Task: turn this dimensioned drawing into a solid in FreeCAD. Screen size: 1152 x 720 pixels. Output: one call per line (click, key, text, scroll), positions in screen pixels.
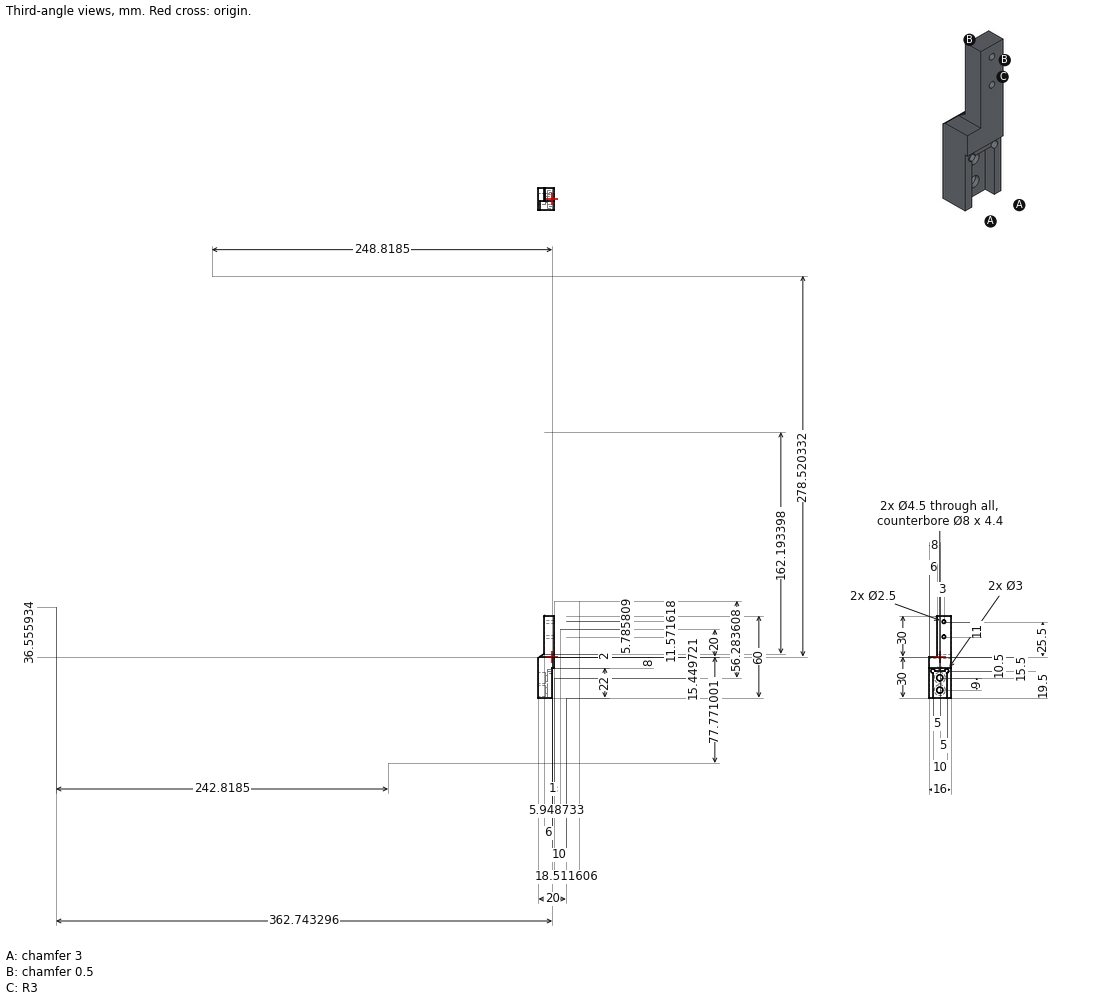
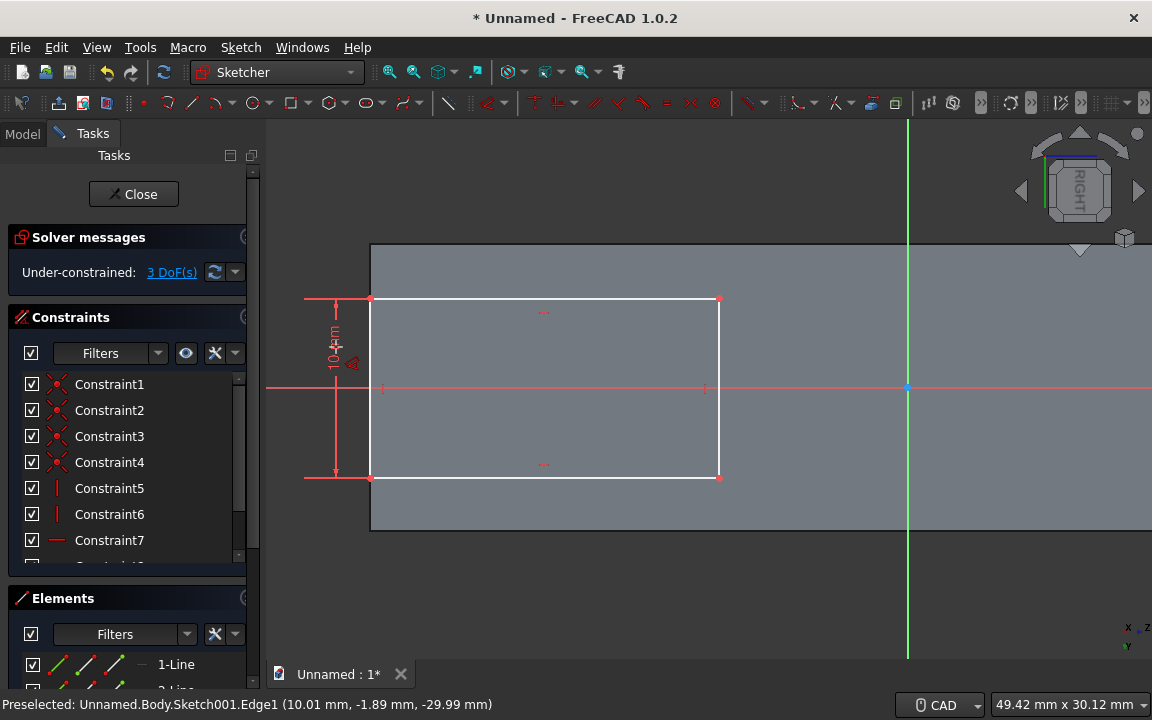
click(370, 299)
click(942, 343)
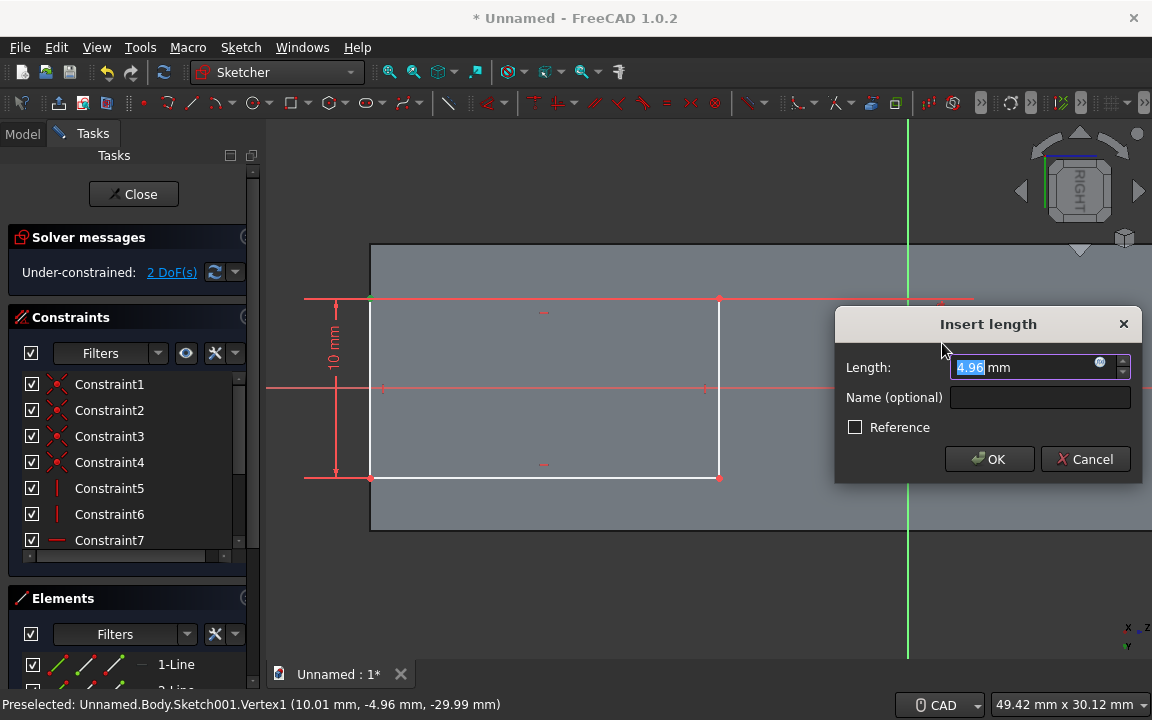
text(5)
key(Return)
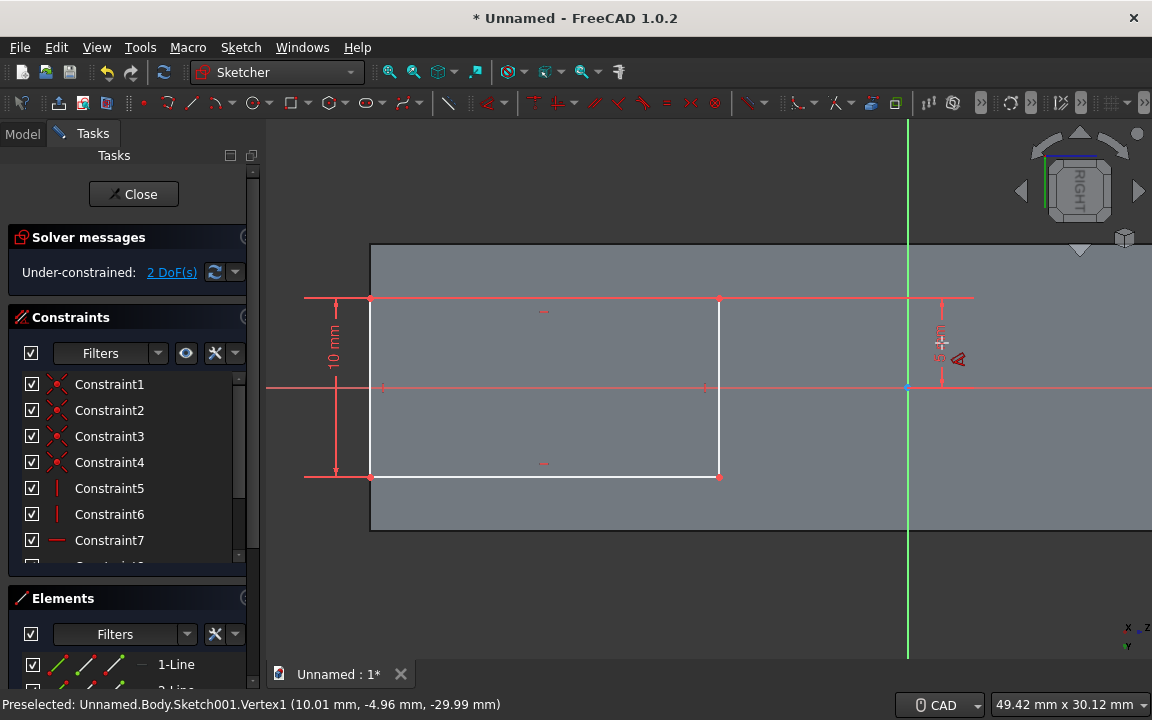
click(370, 298)
click(639, 264)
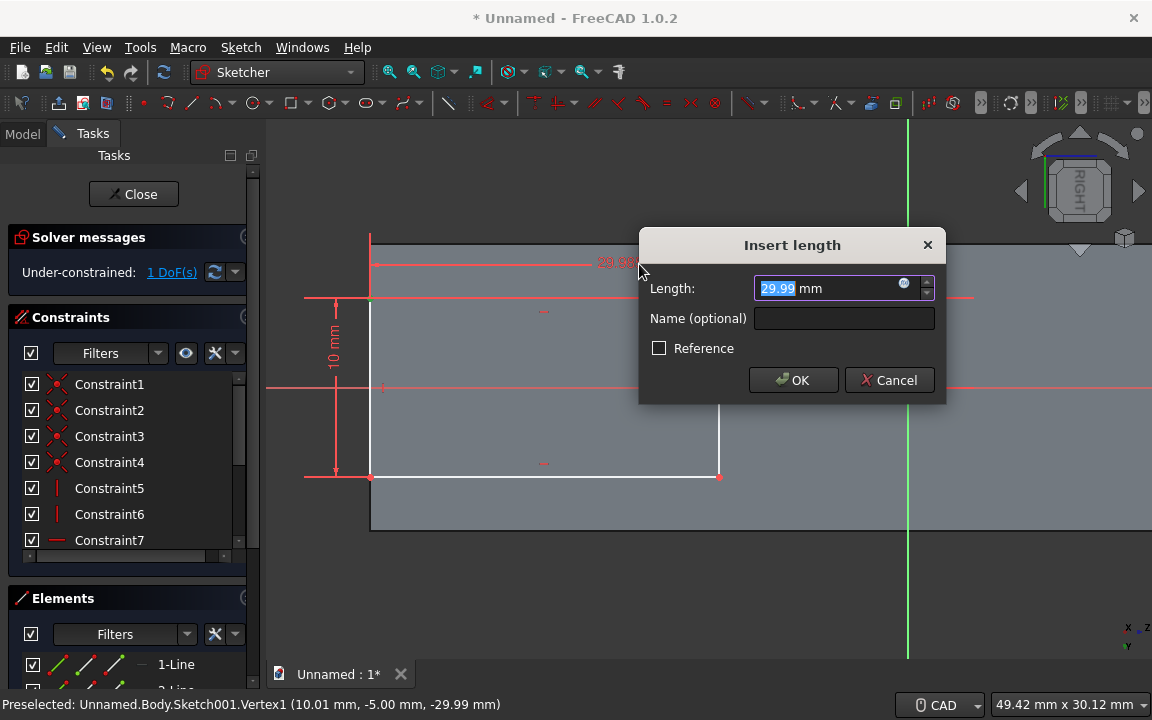
text(30)
key(Return)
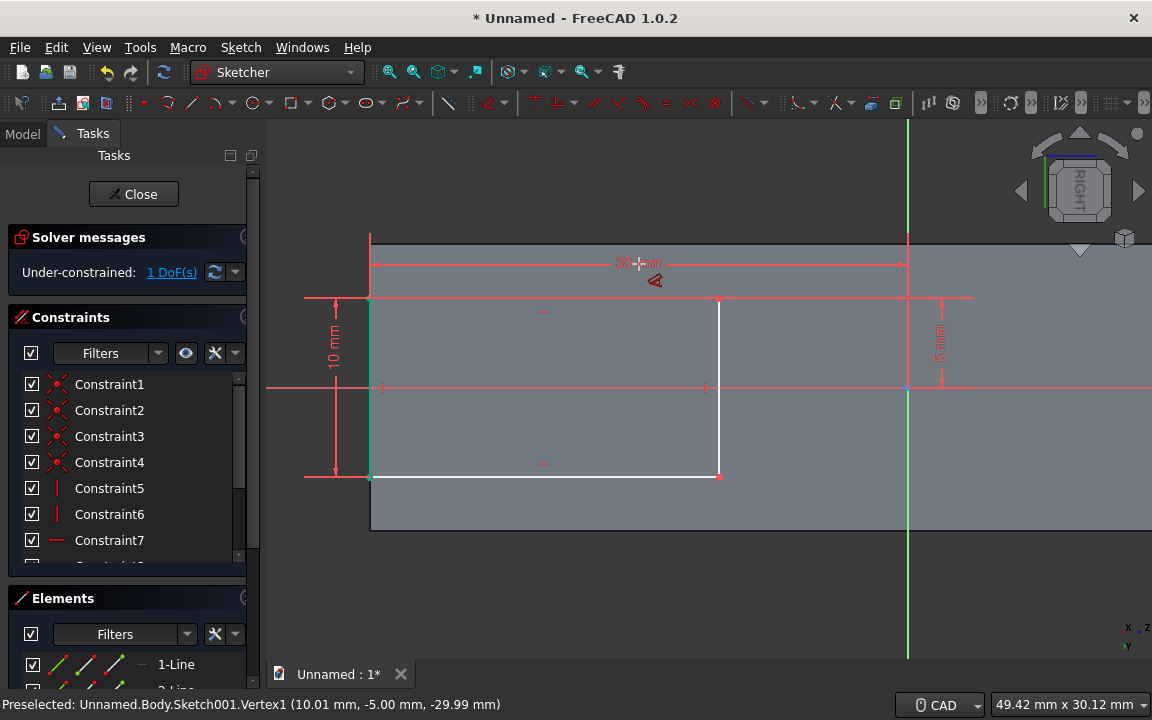
click(475, 477)
click(544, 511)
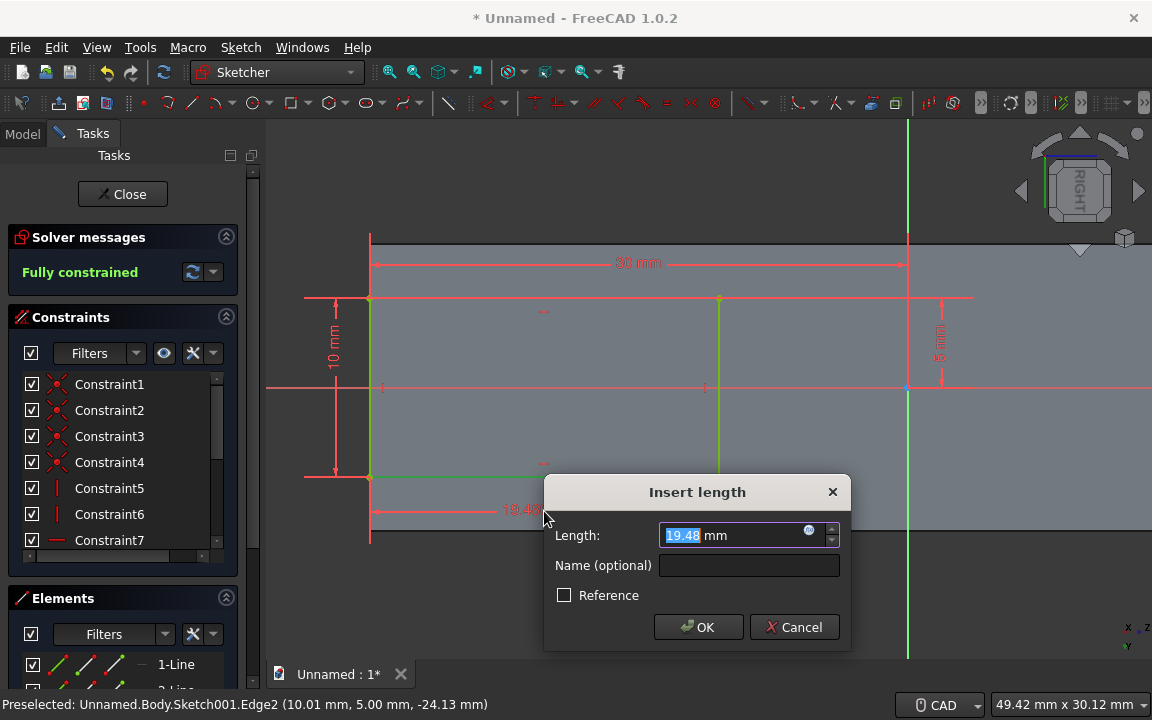
text(19.5)
key(Return)
key(Escape)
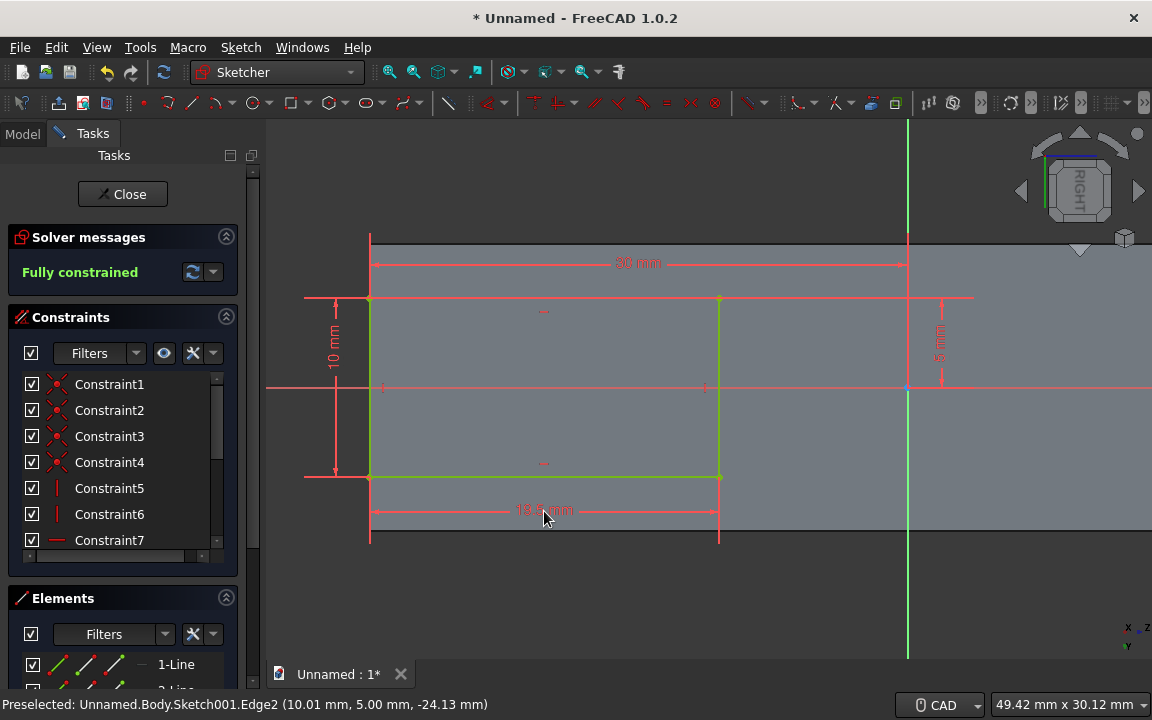
click(123, 194)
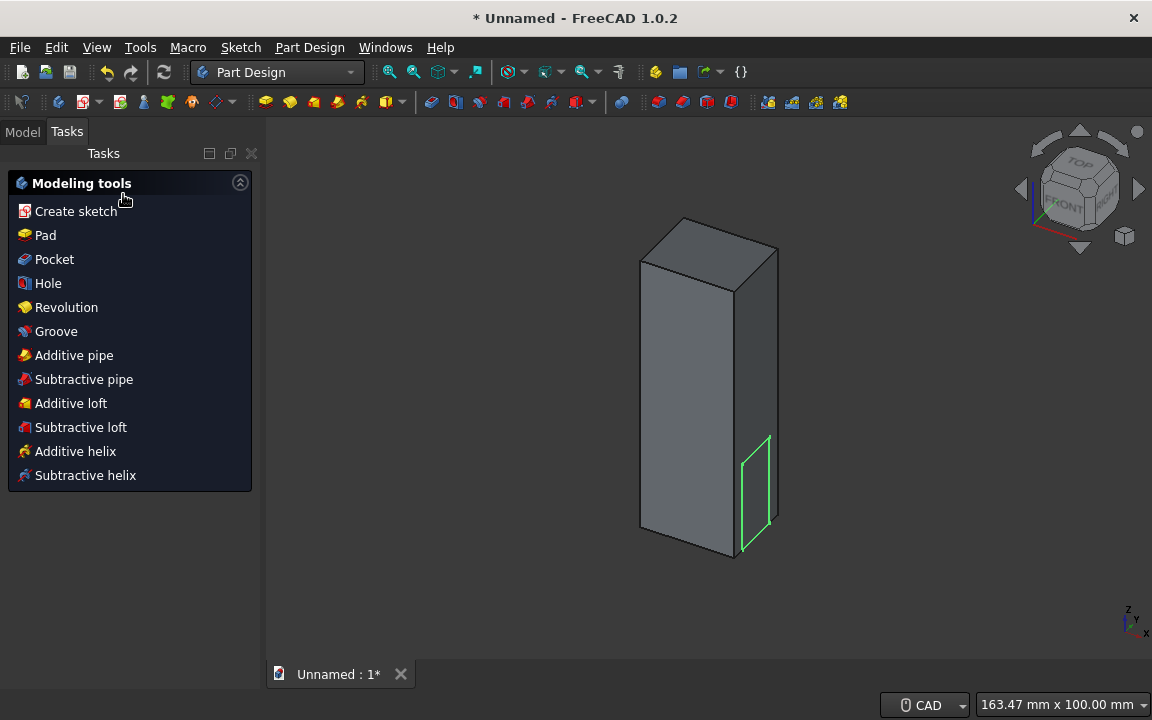
click(432, 102)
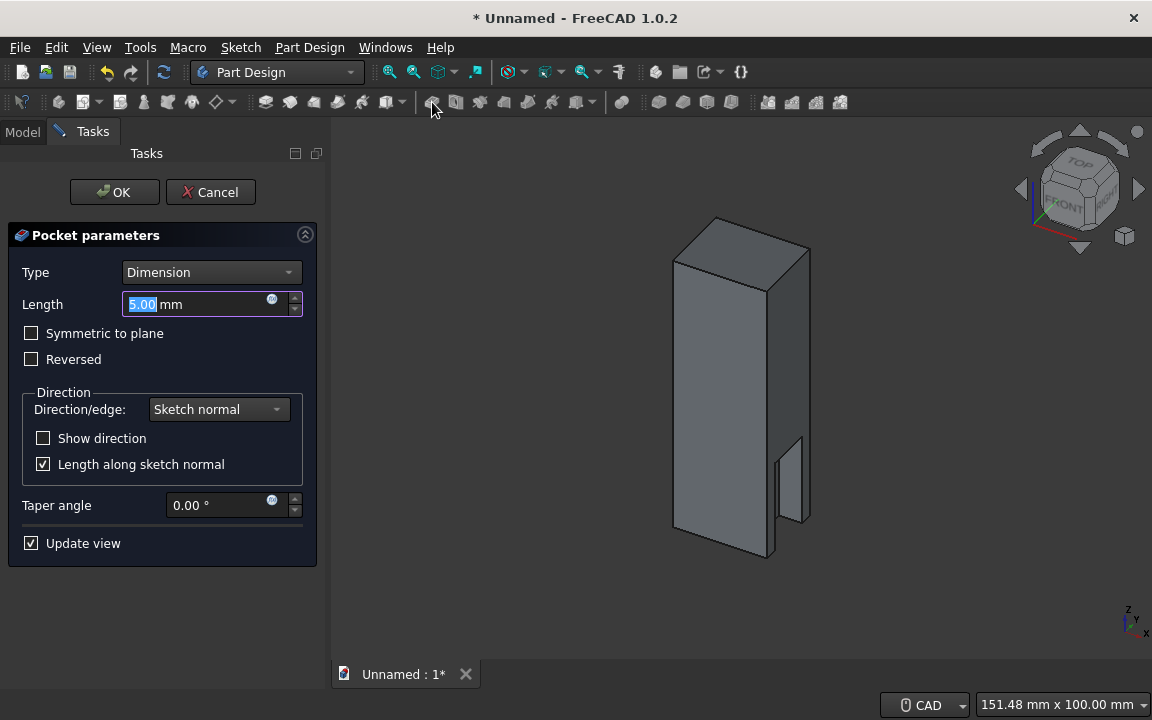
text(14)
key(Tab)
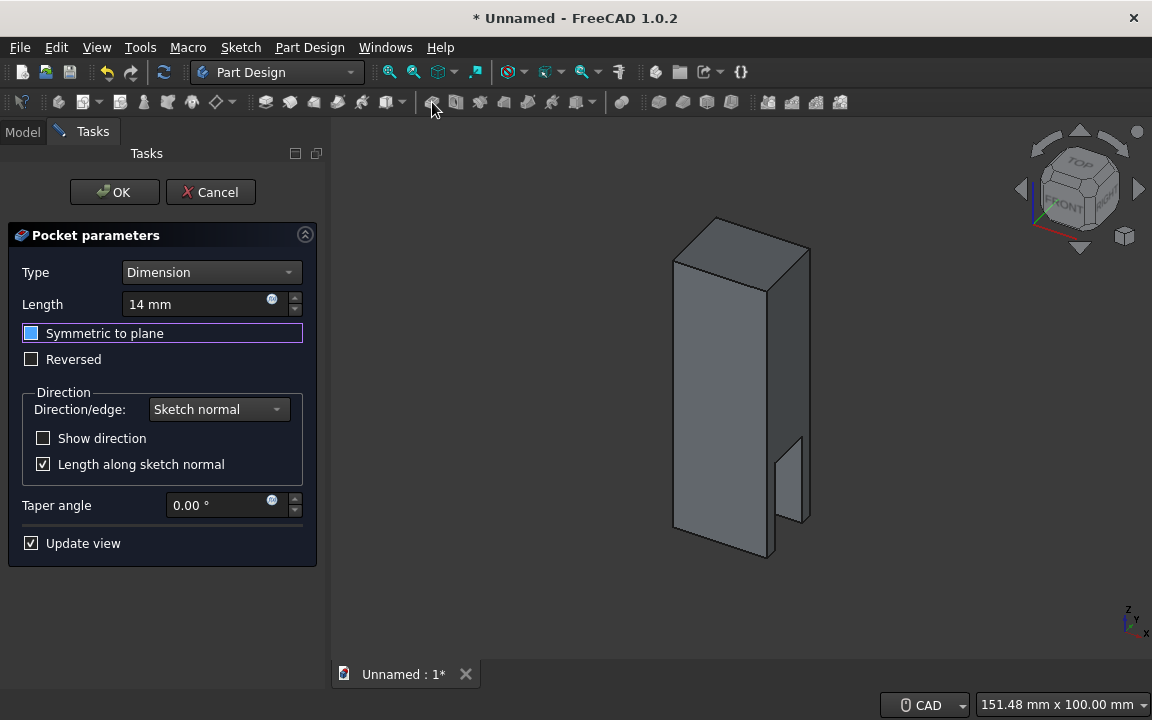
click(115, 192)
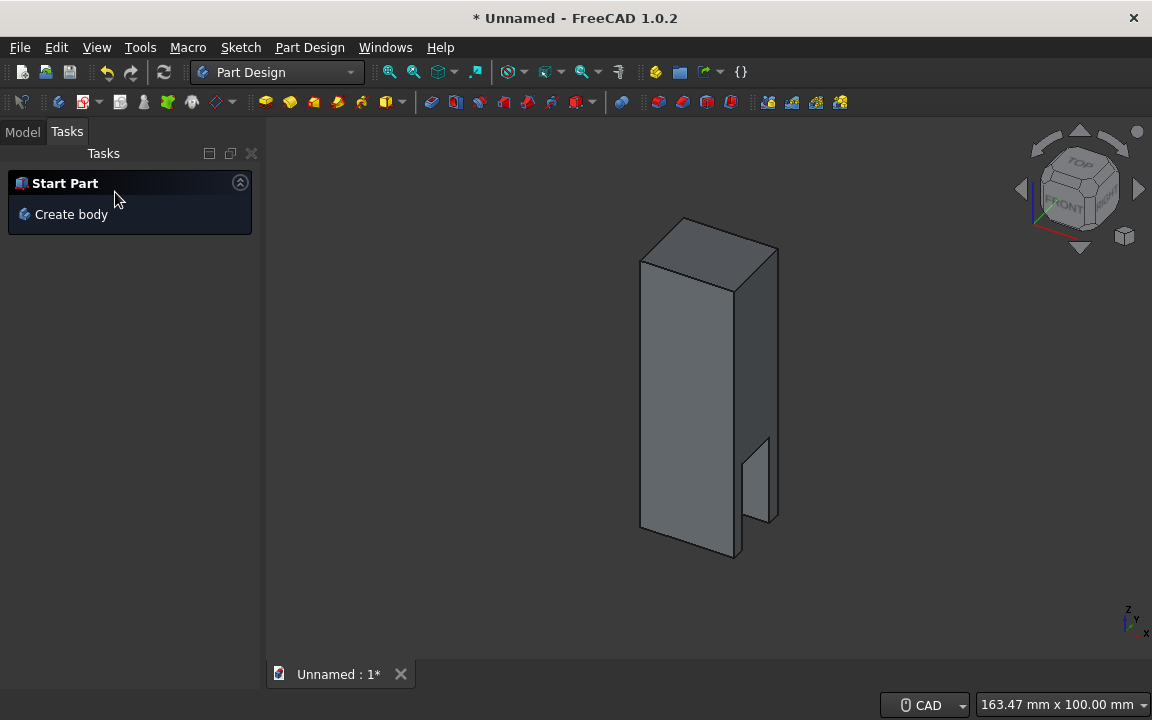
scroll(738, 553, up, 5)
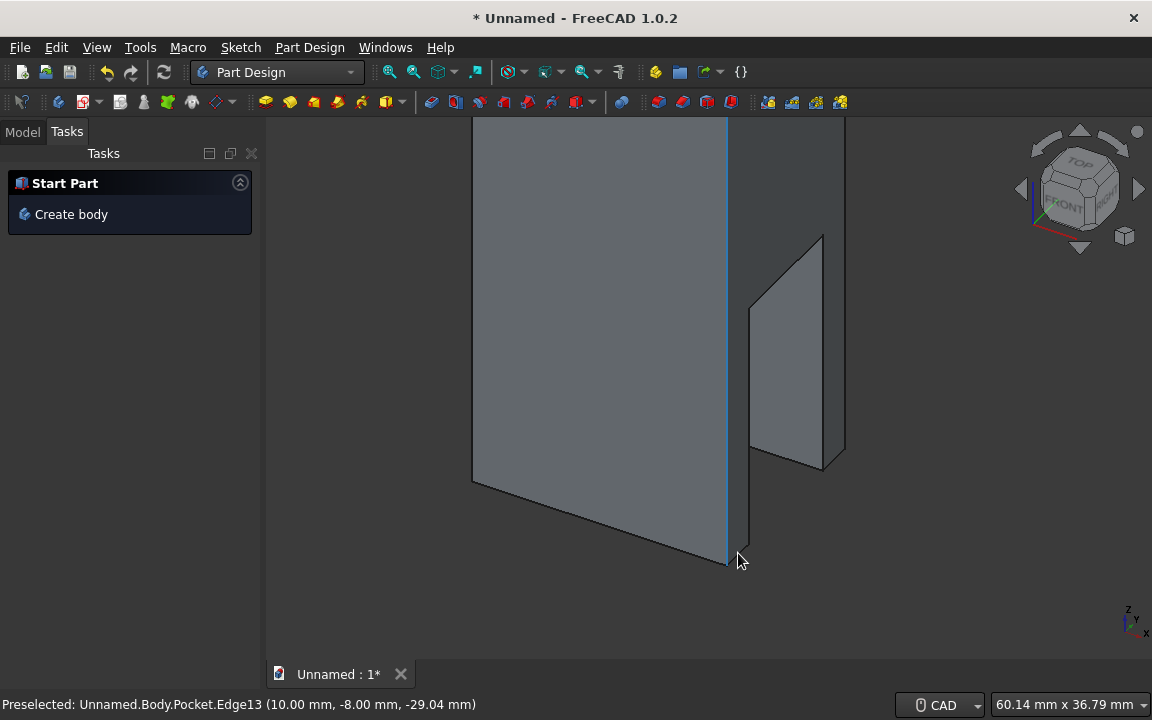
click(390, 72)